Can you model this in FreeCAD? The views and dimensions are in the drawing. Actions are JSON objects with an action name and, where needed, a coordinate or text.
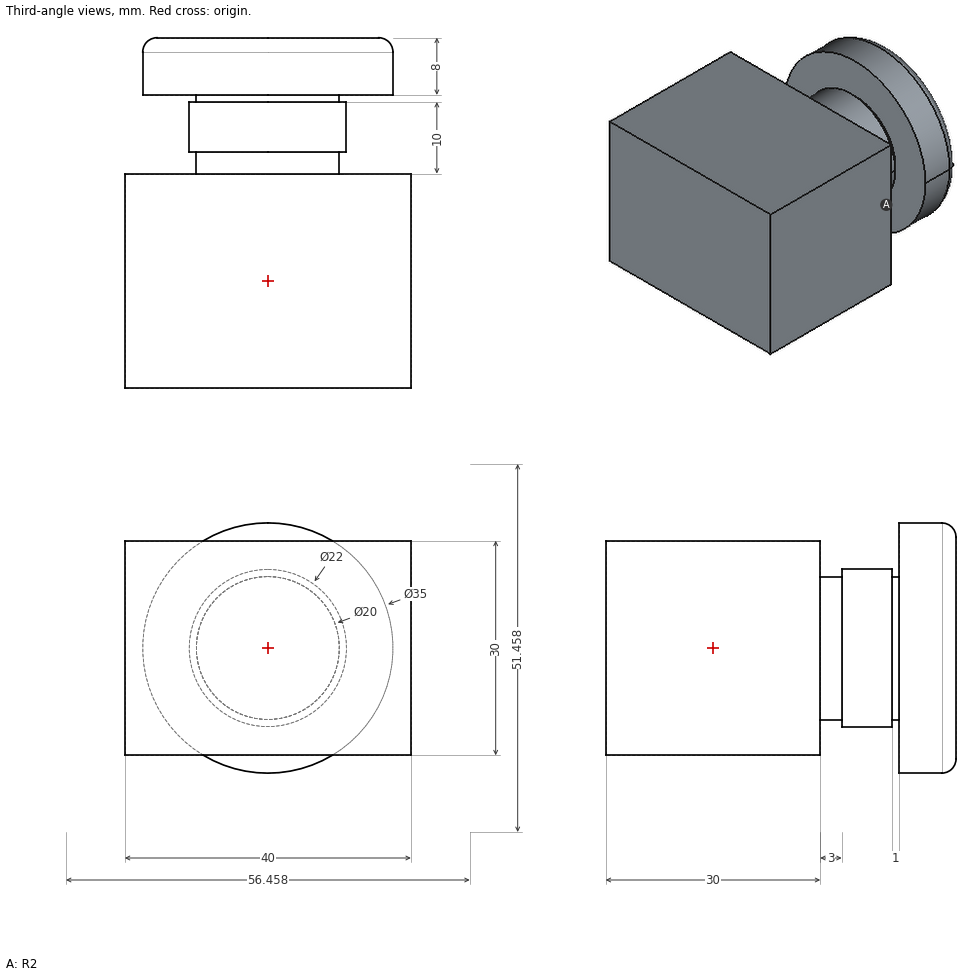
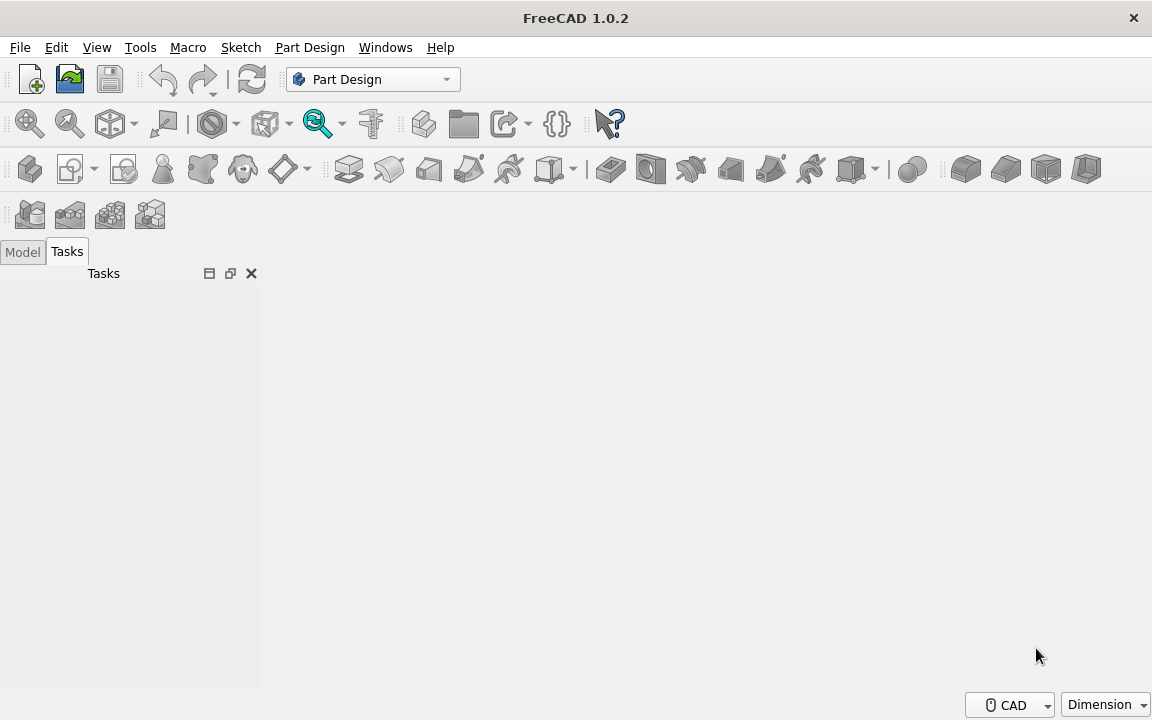
{"action": "left_click", "coordinate": [30, 80]}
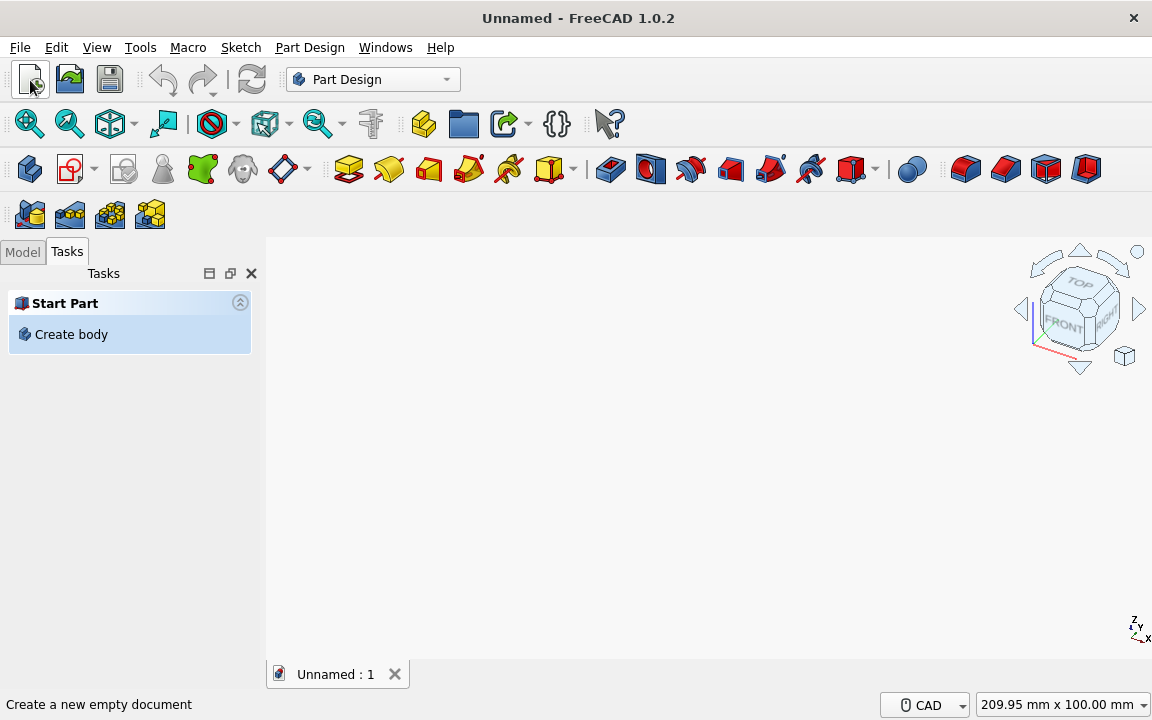
{"action": "left_click", "coordinate": [70, 170]}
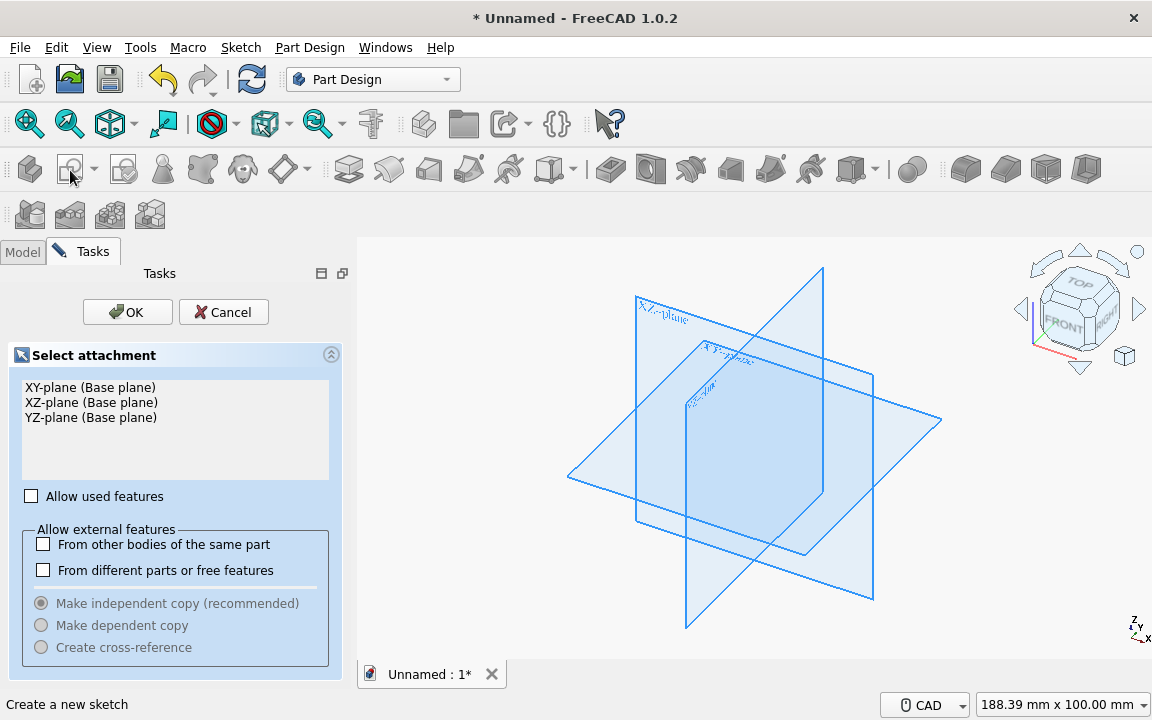
{"action": "left_click", "coordinate": [82, 402]}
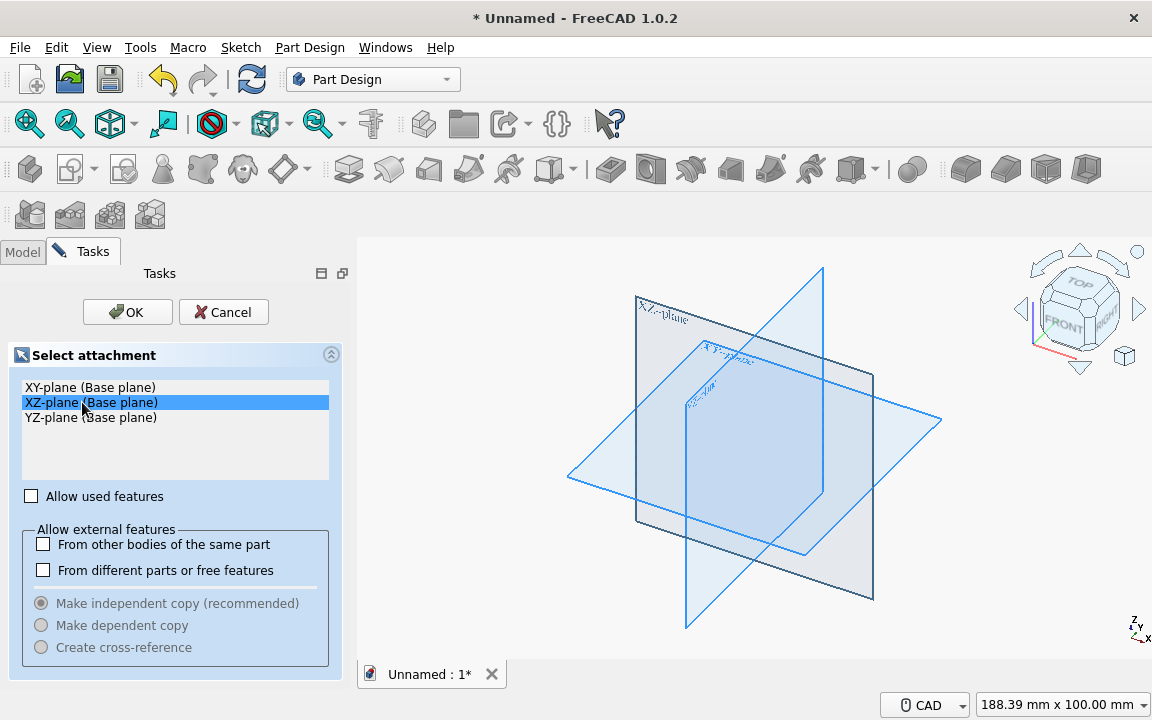
{"action": "left_click", "coordinate": [128, 312]}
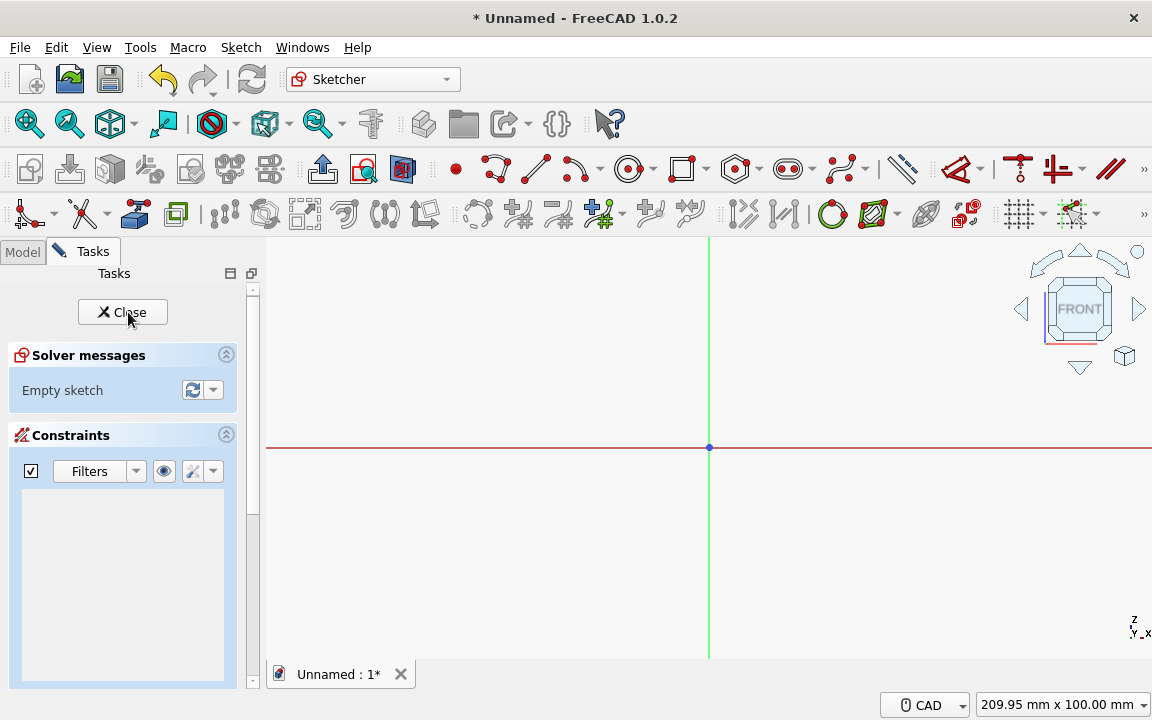
{"action": "scroll", "coordinate": [765, 448], "scroll_direction": "up", "scroll_amount": 4}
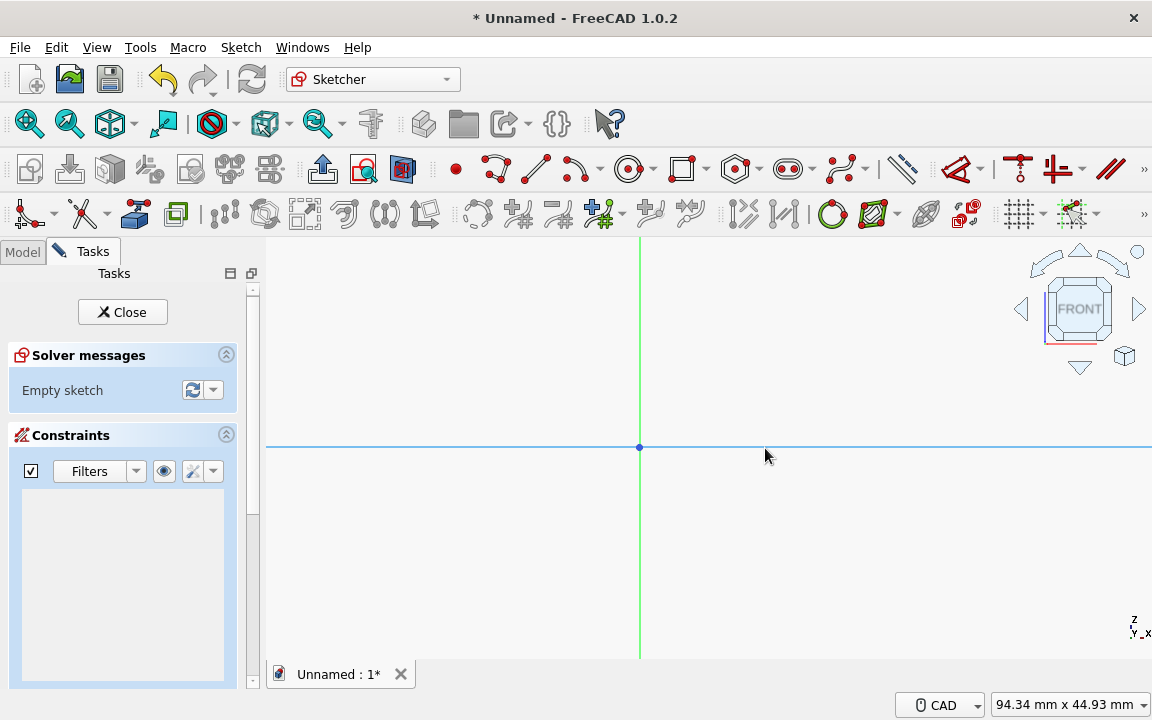
{"action": "key", "text": "g v"}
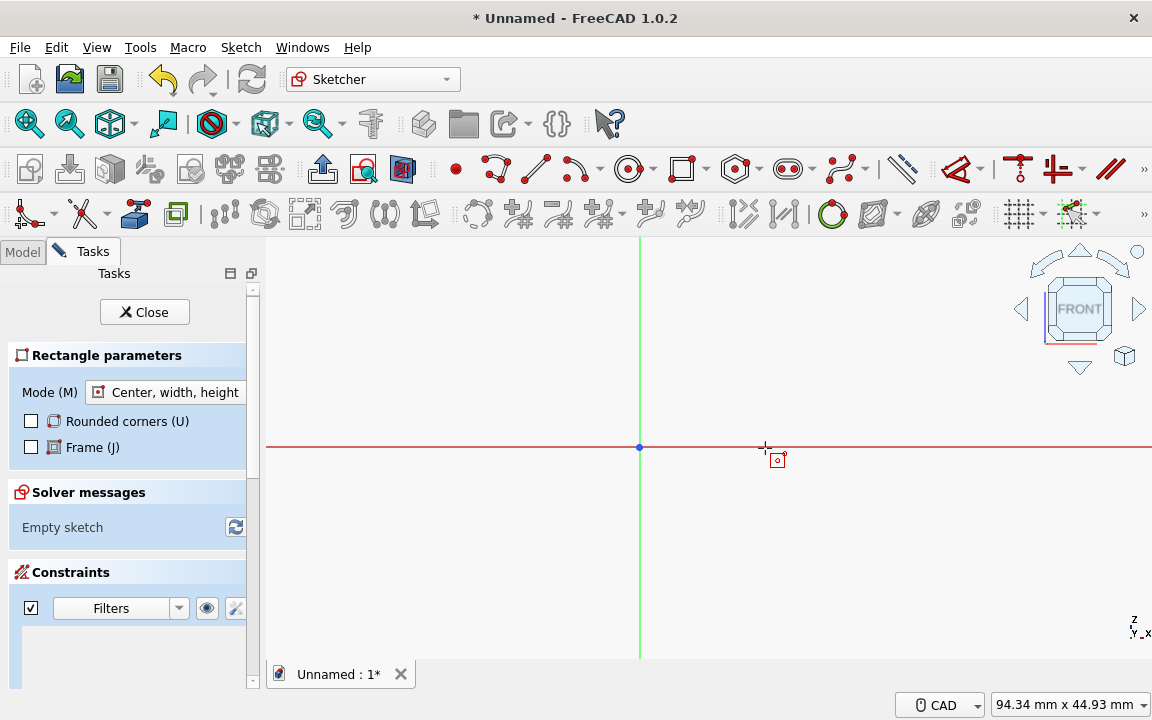
{"action": "left_click", "coordinate": [640, 447]}
{"action": "mouse_move", "coordinate": [828, 307]}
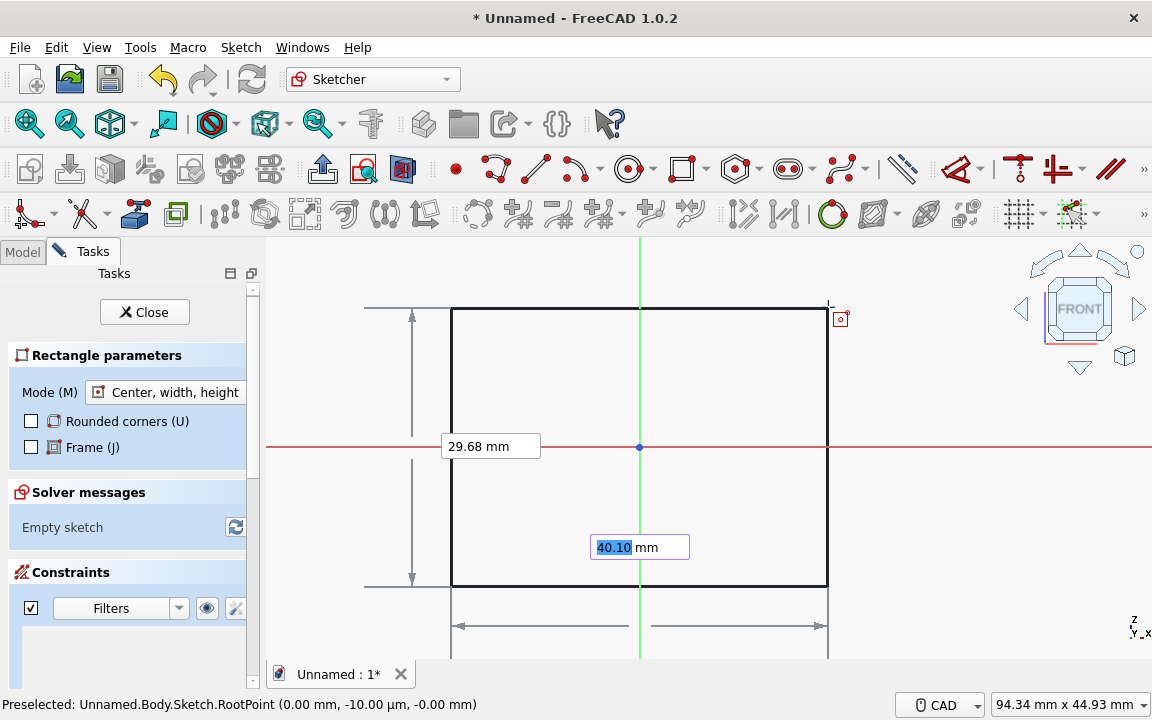
{"action": "type", "text": "40"}
{"action": "key", "text": "Tab"}
{"action": "type", "text": "30"}
{"action": "key", "text": "Return"}
{"action": "key", "text": "Escape"}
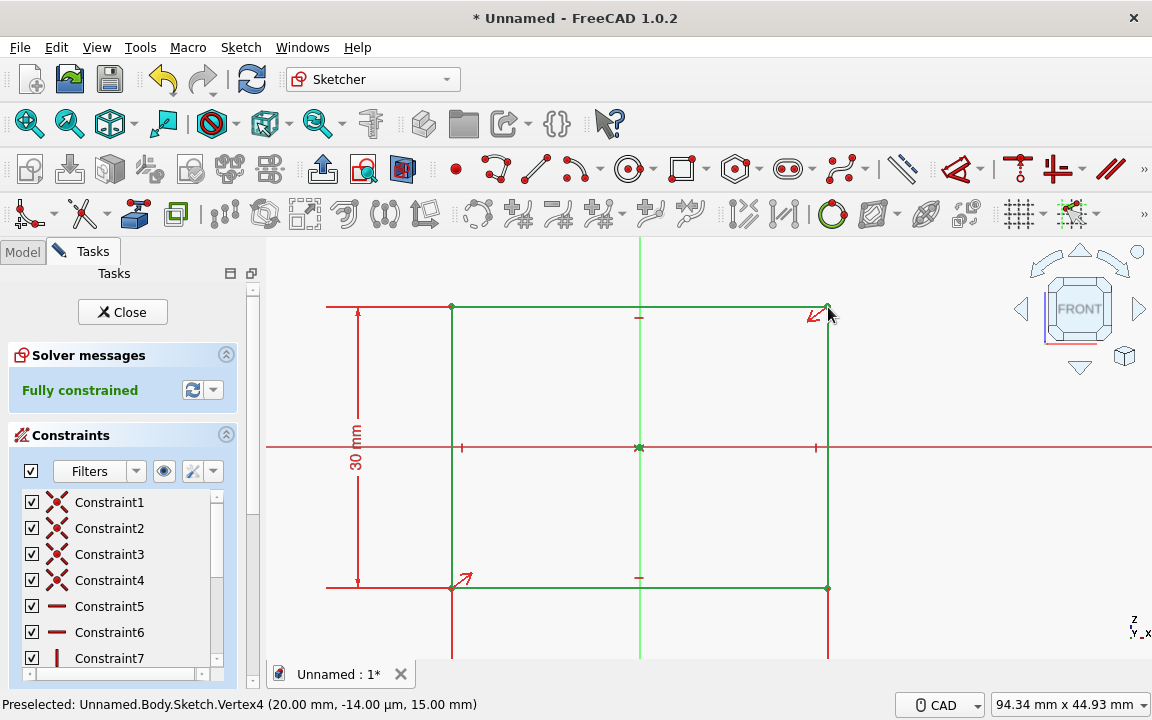
{"action": "left_click", "coordinate": [123, 312]}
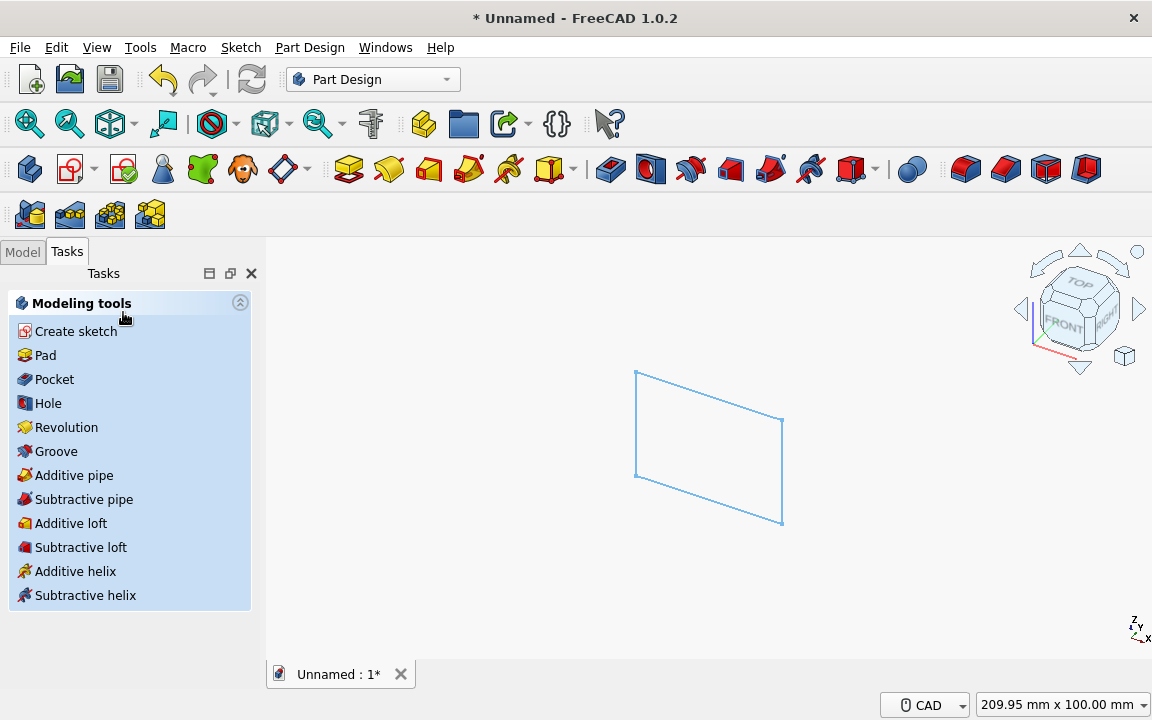
{"action": "left_click", "coordinate": [350, 170]}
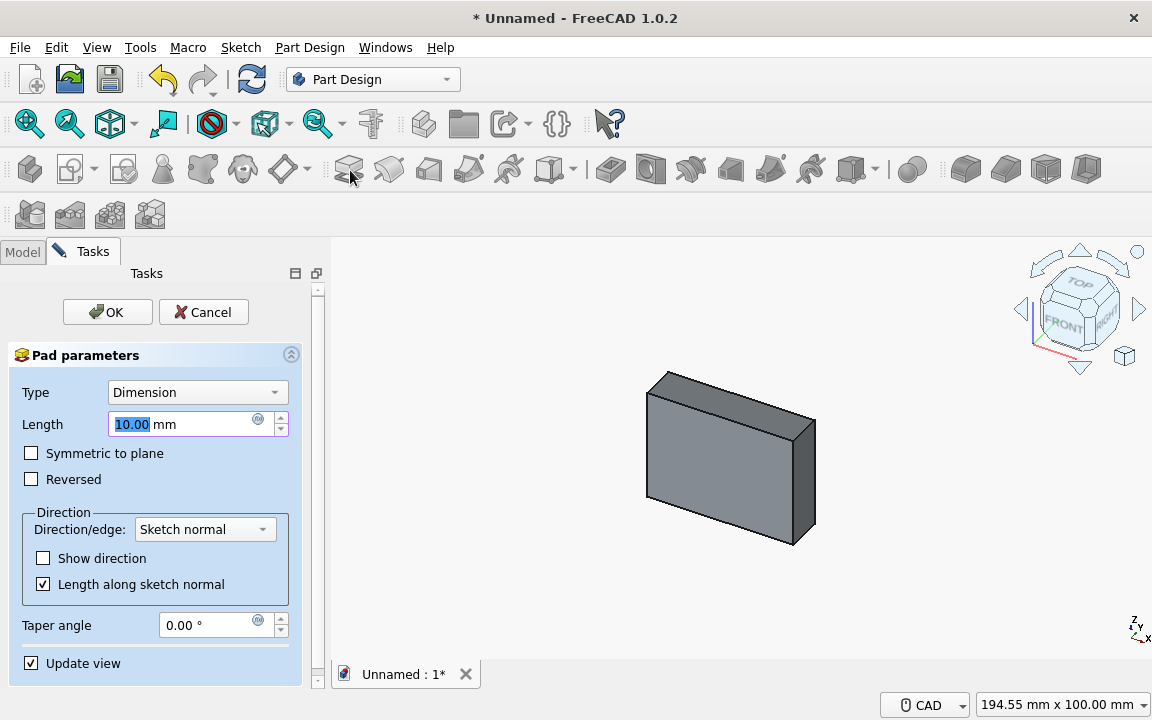
{"action": "type", "text": "30"}
{"action": "key", "text": "Tab"}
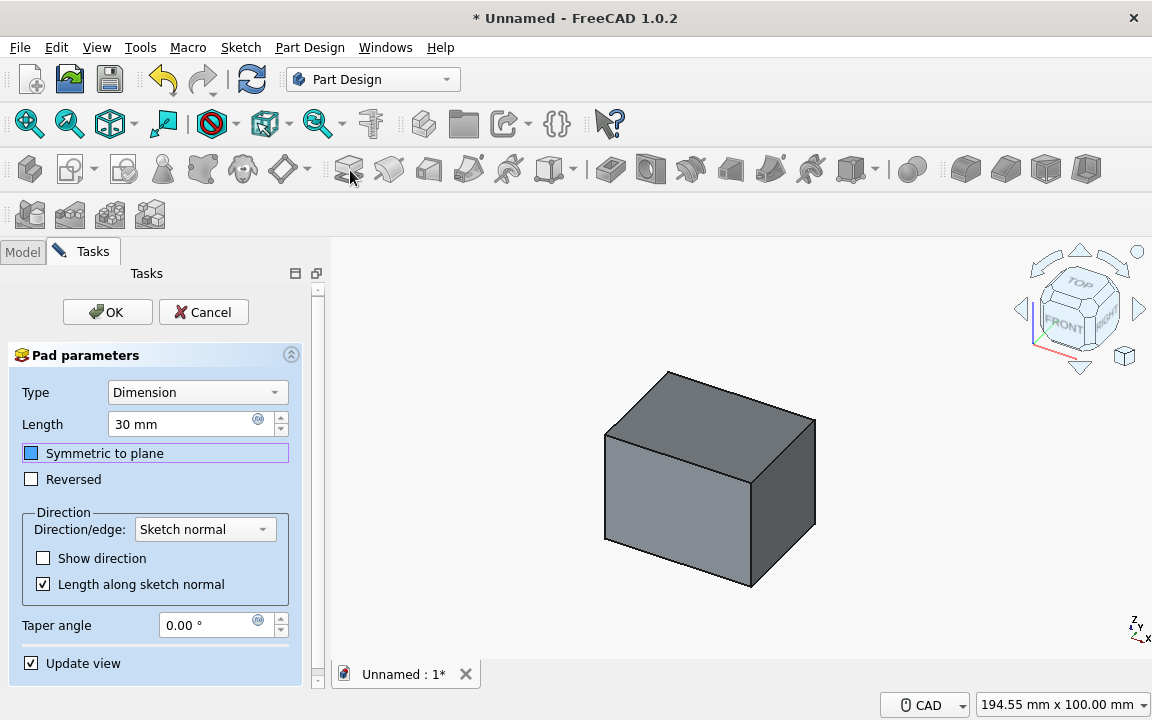
{"action": "left_click", "coordinate": [30, 453]}